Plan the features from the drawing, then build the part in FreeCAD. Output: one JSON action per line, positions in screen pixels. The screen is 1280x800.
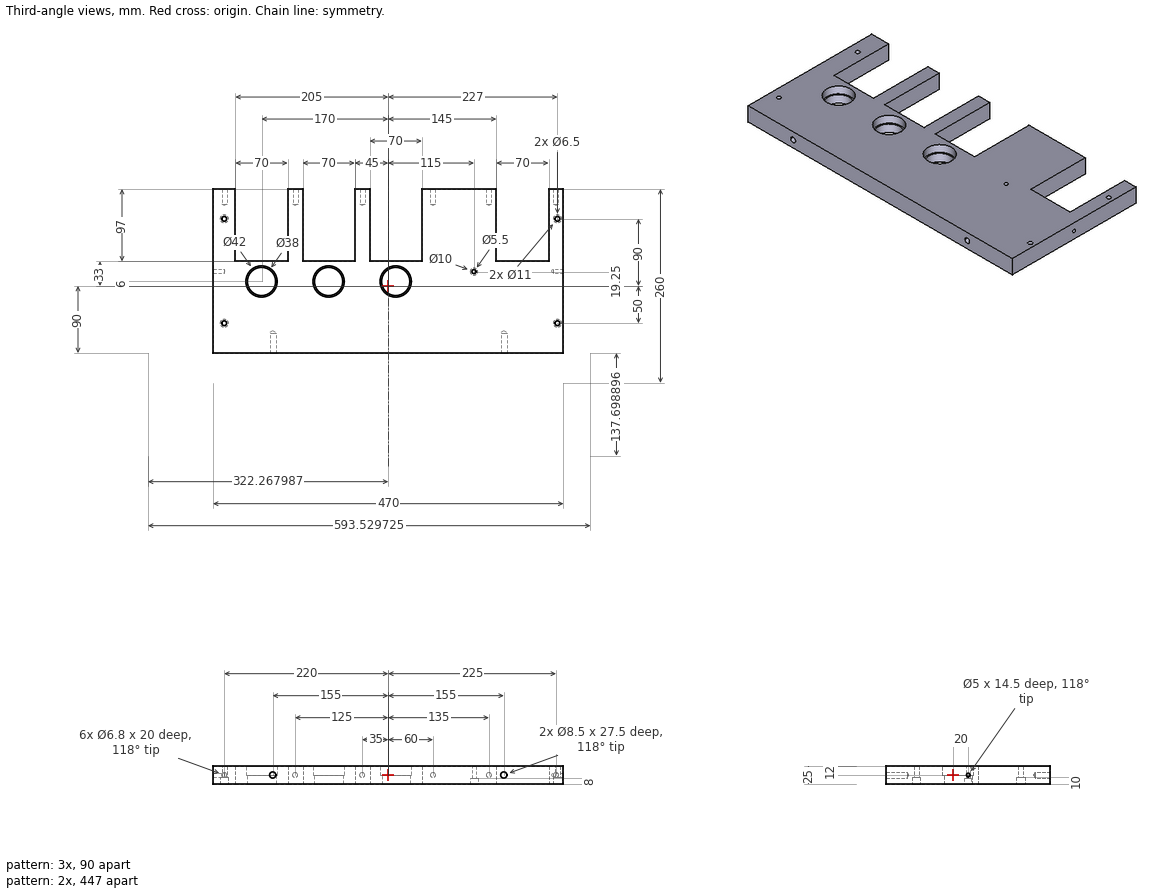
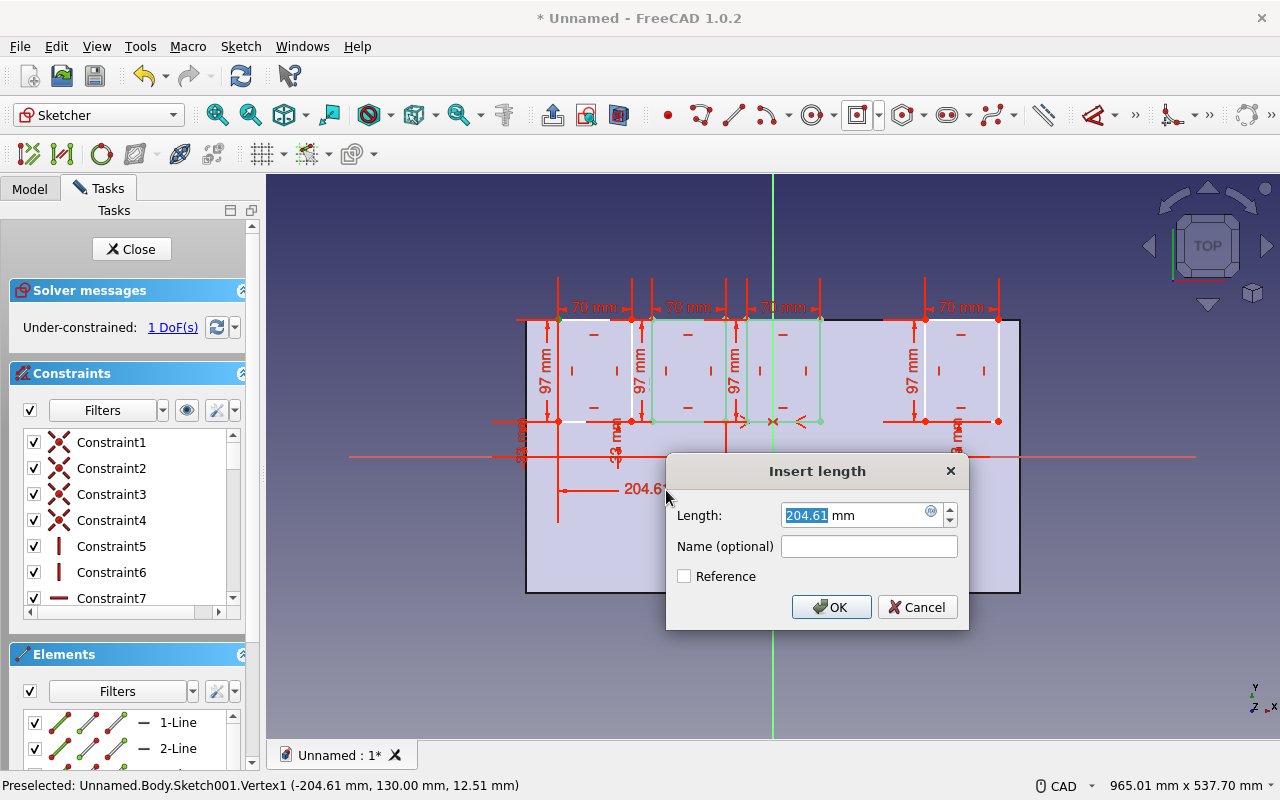
{"action": "type", "text": "205"}
{"action": "key", "text": "Return"}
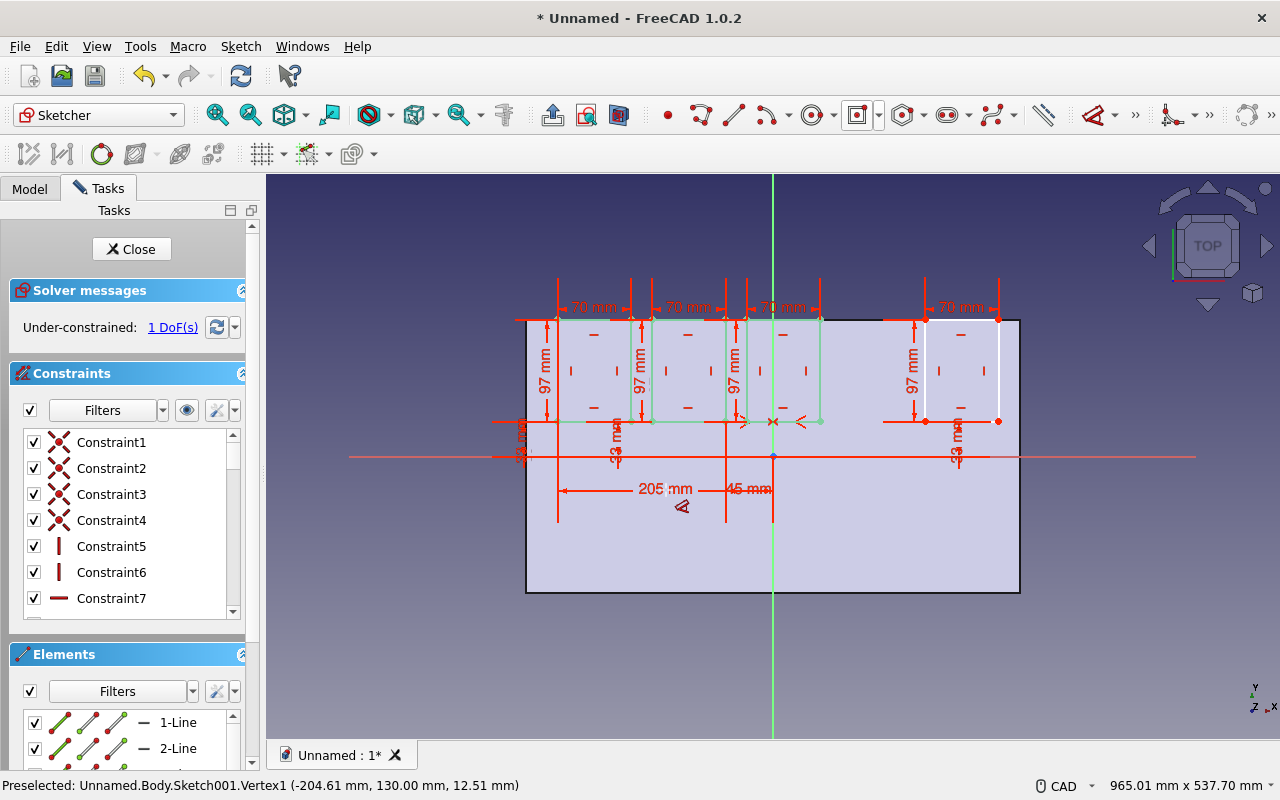
{"action": "left_click", "coordinate": [925, 320]}
{"action": "left_click", "coordinate": [849, 490]}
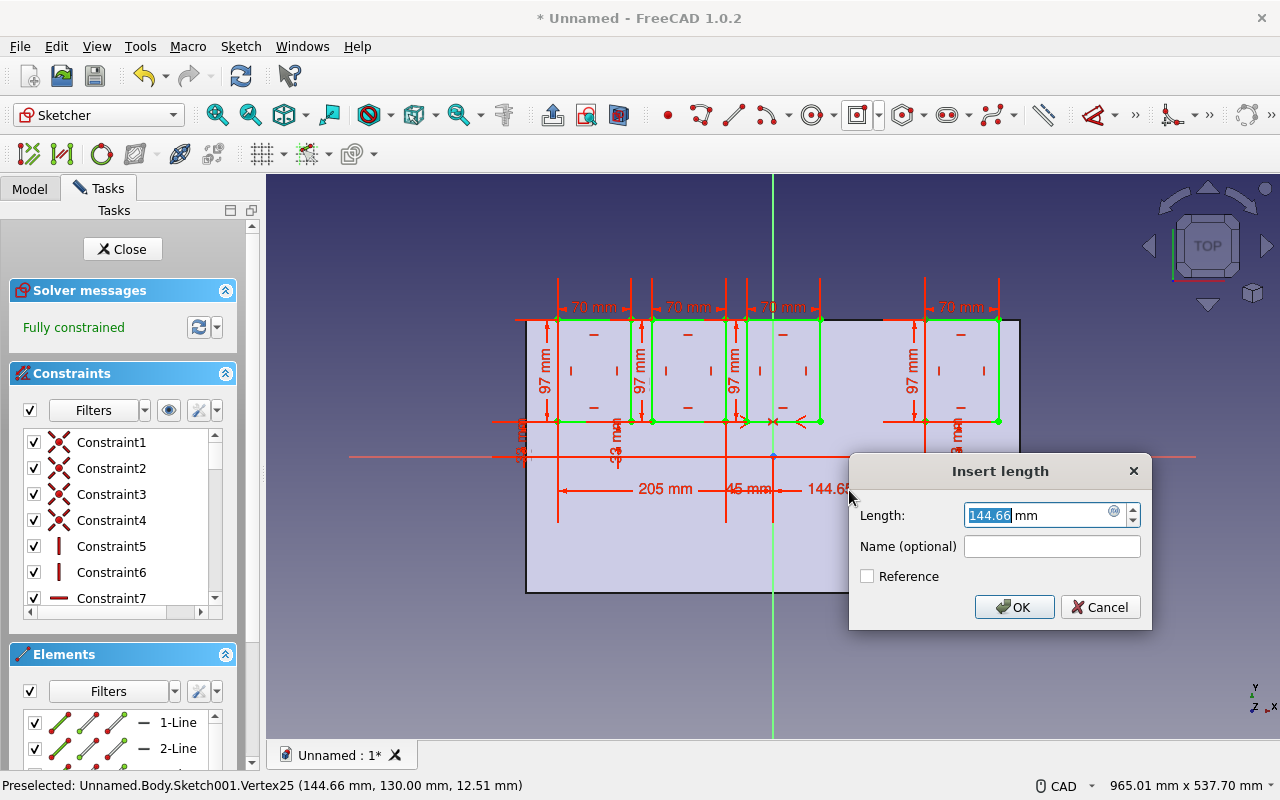
{"action": "type", "text": "145"}
{"action": "key", "text": "Return"}
{"action": "key", "text": "Escape"}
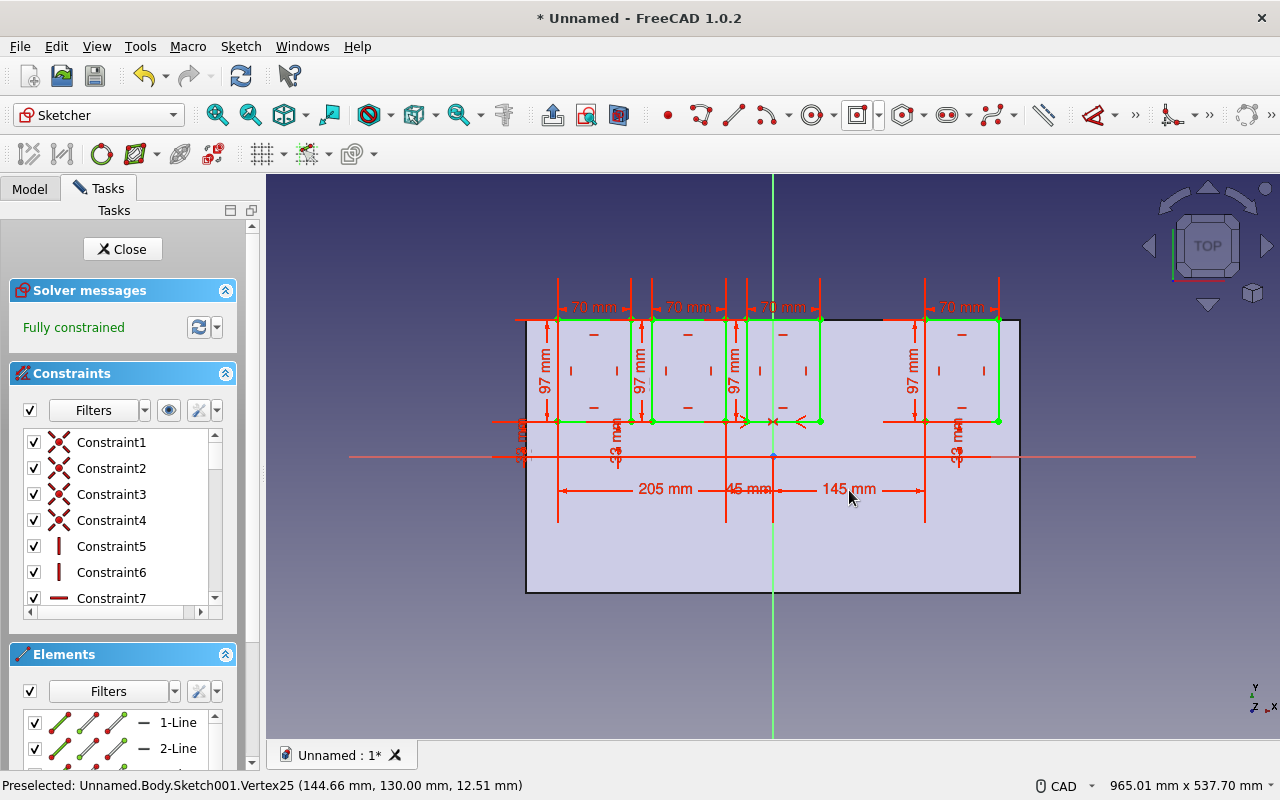
{"action": "left_click", "coordinate": [123, 249]}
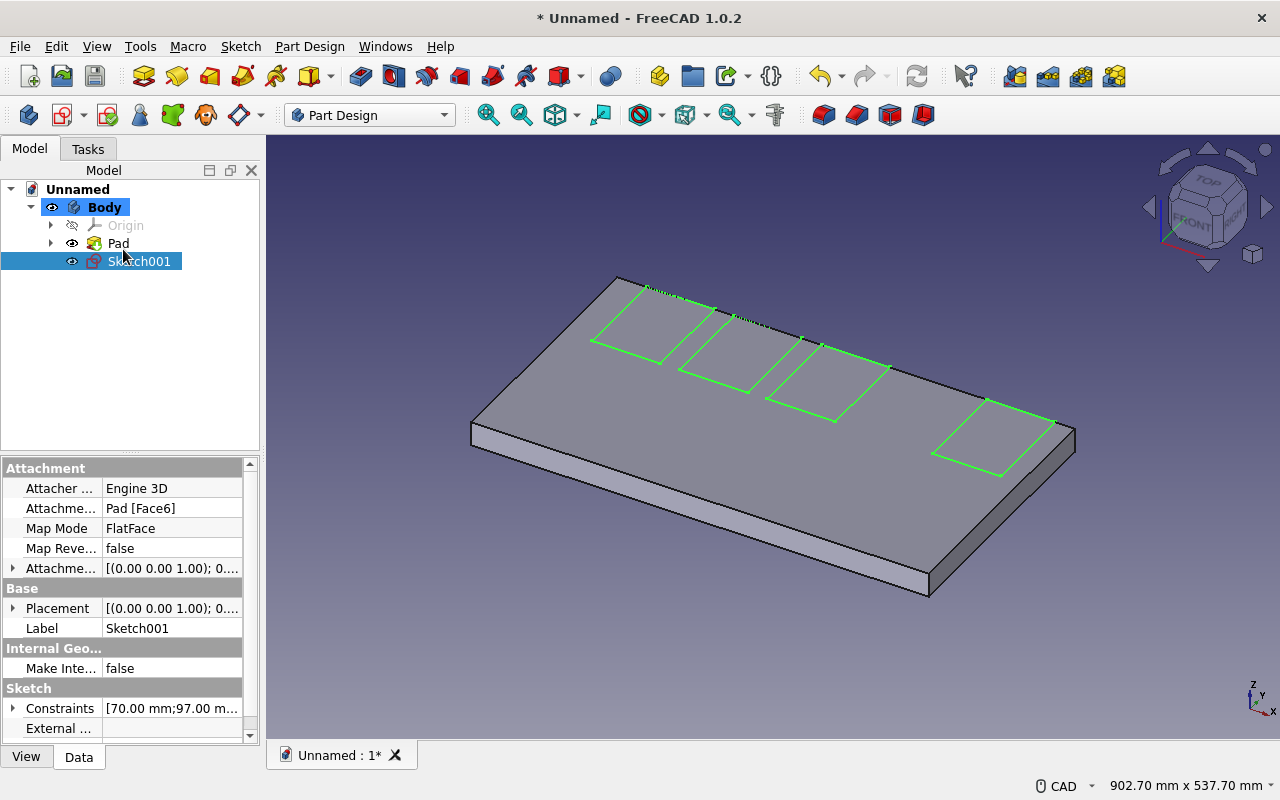
{"action": "left_click", "coordinate": [361, 76]}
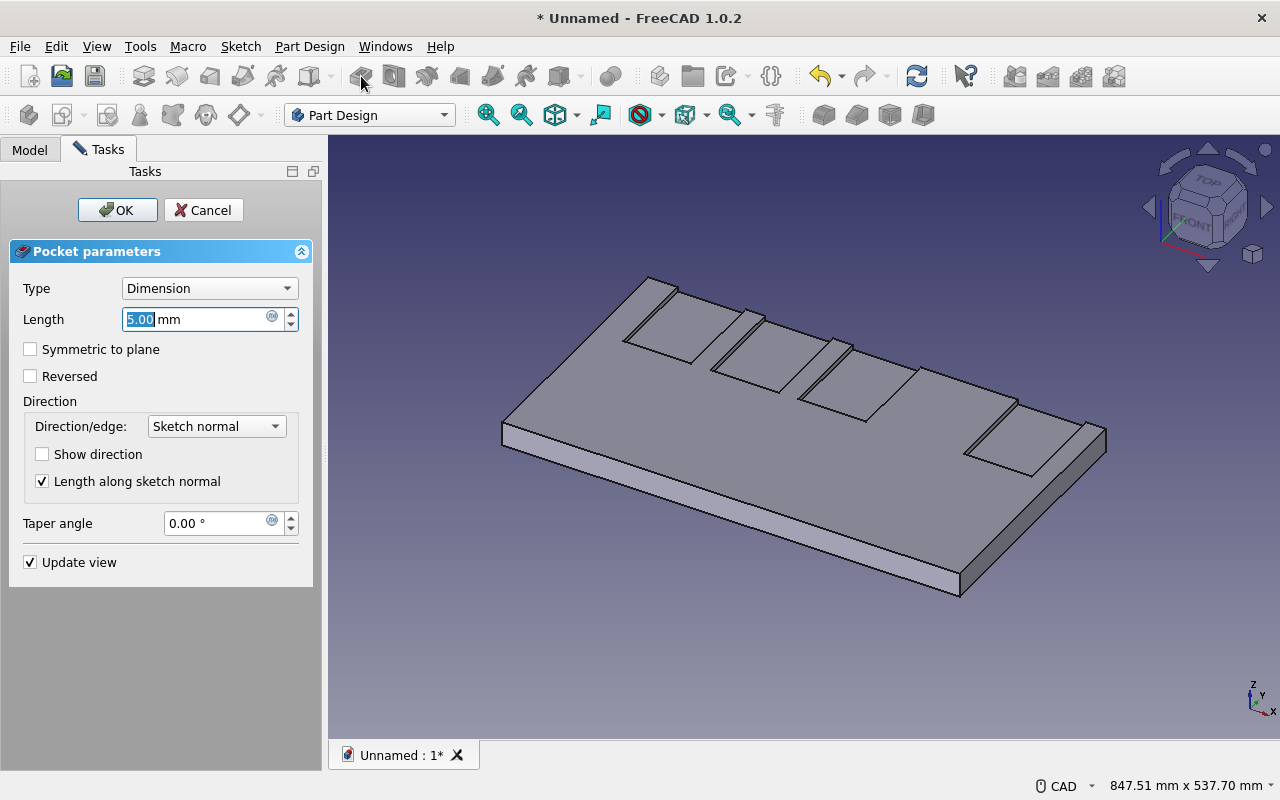
{"action": "type", "text": "97"}
{"action": "key", "text": "Tab"}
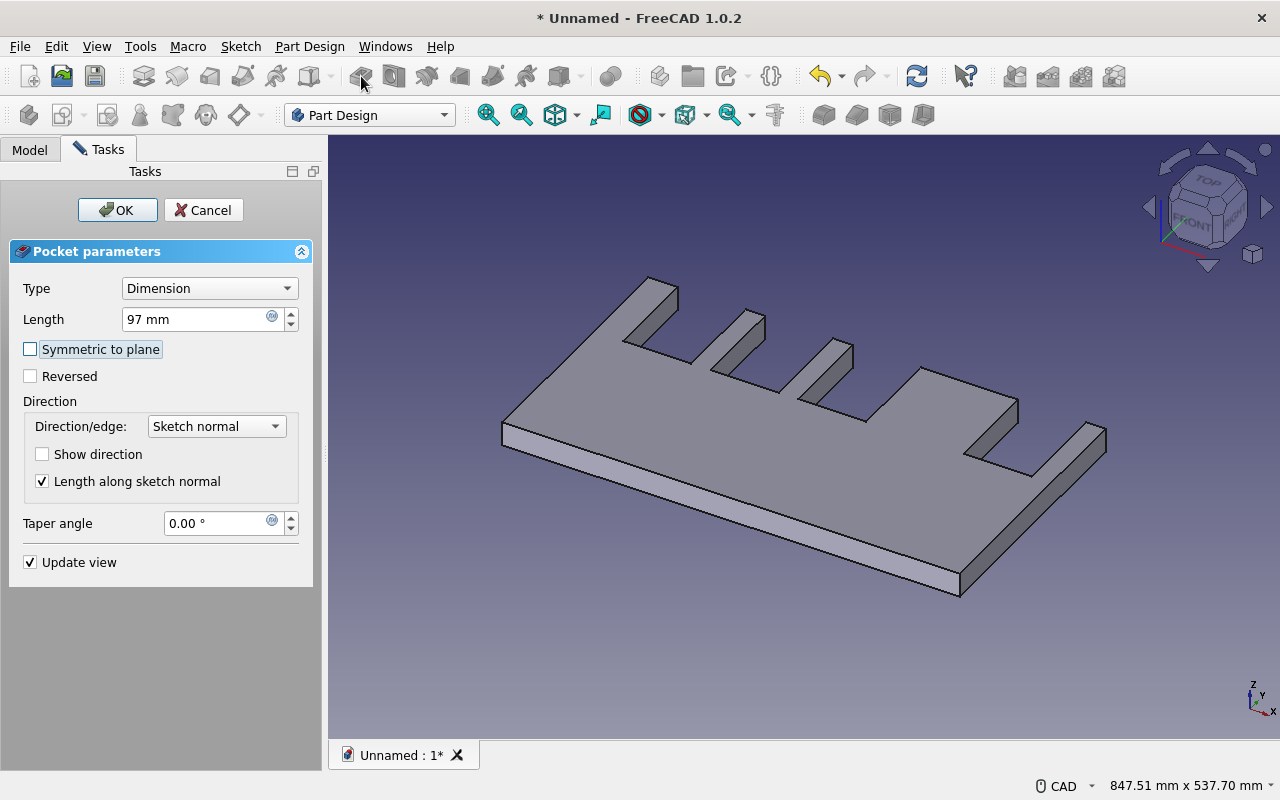
{"action": "left_click", "coordinate": [118, 210]}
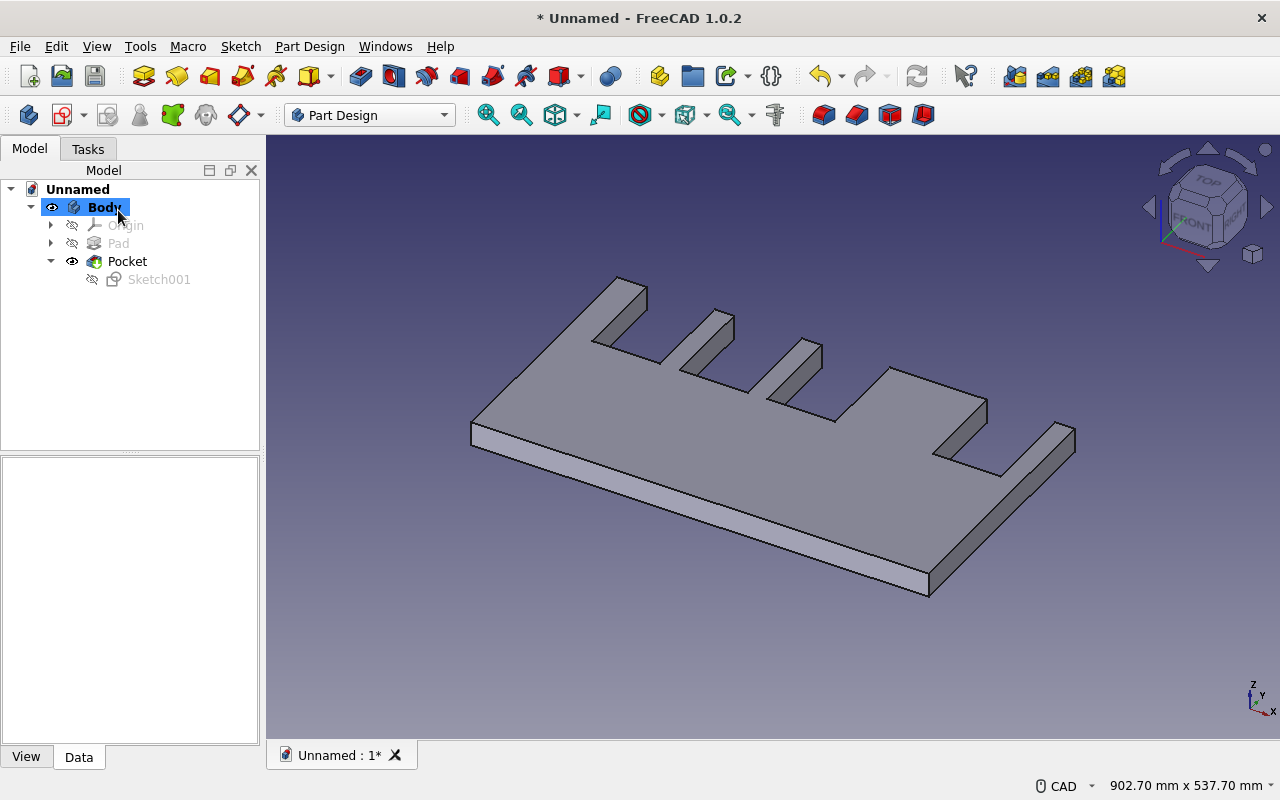
{"action": "left_click", "coordinate": [817, 467]}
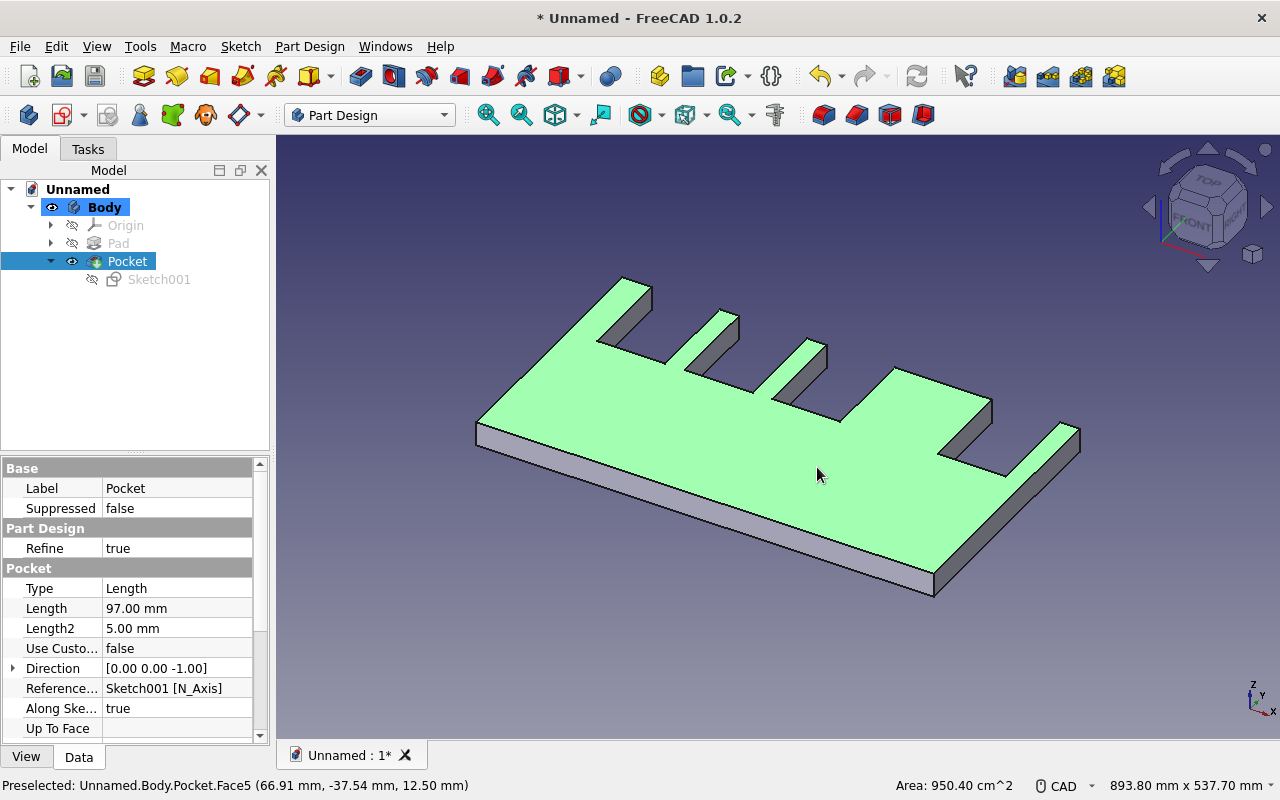
{"action": "left_click", "coordinate": [62, 116]}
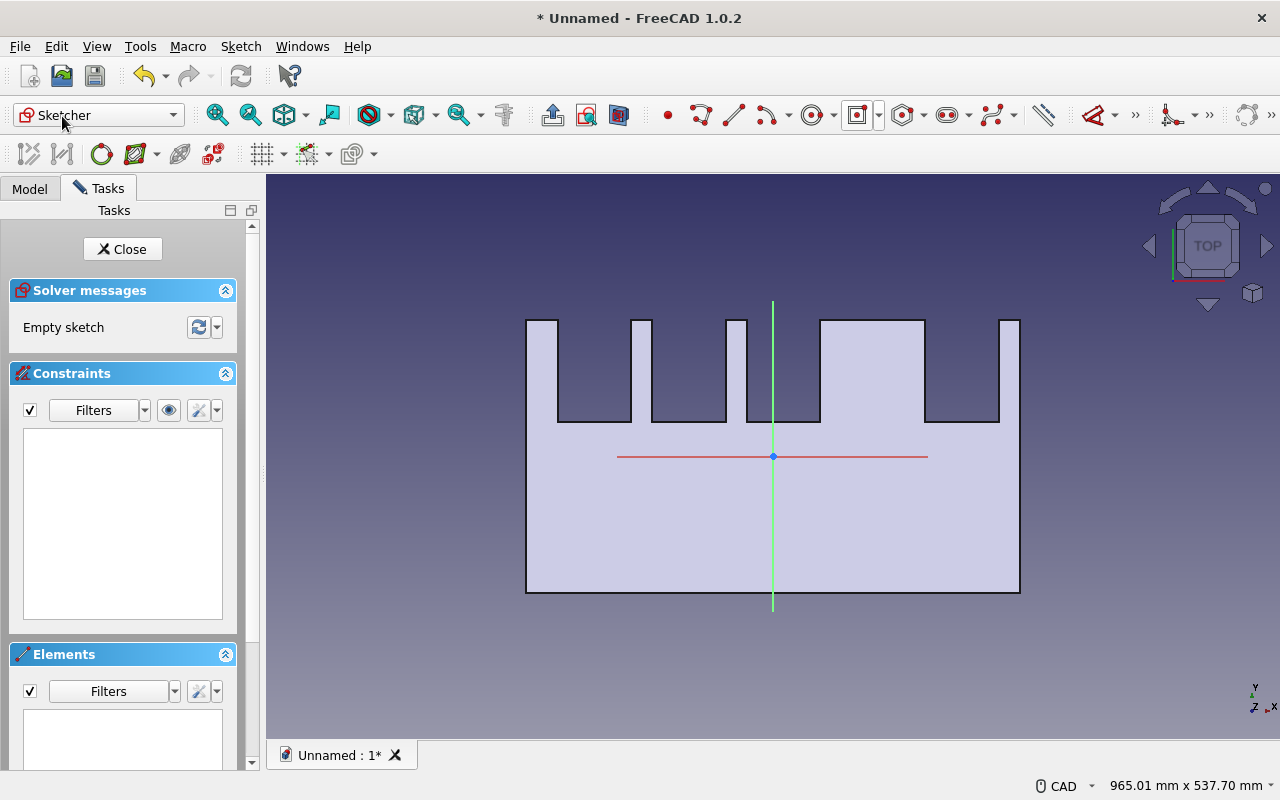
{"action": "scroll", "coordinate": [904, 435], "scroll_direction": "up", "scroll_amount": 15}